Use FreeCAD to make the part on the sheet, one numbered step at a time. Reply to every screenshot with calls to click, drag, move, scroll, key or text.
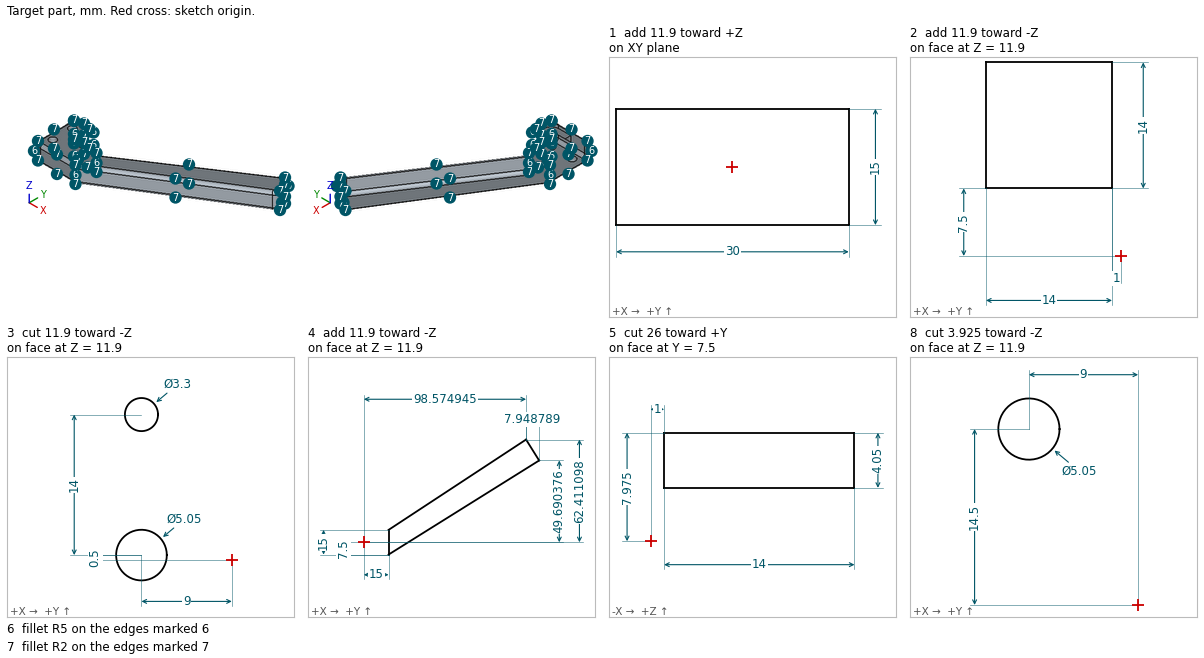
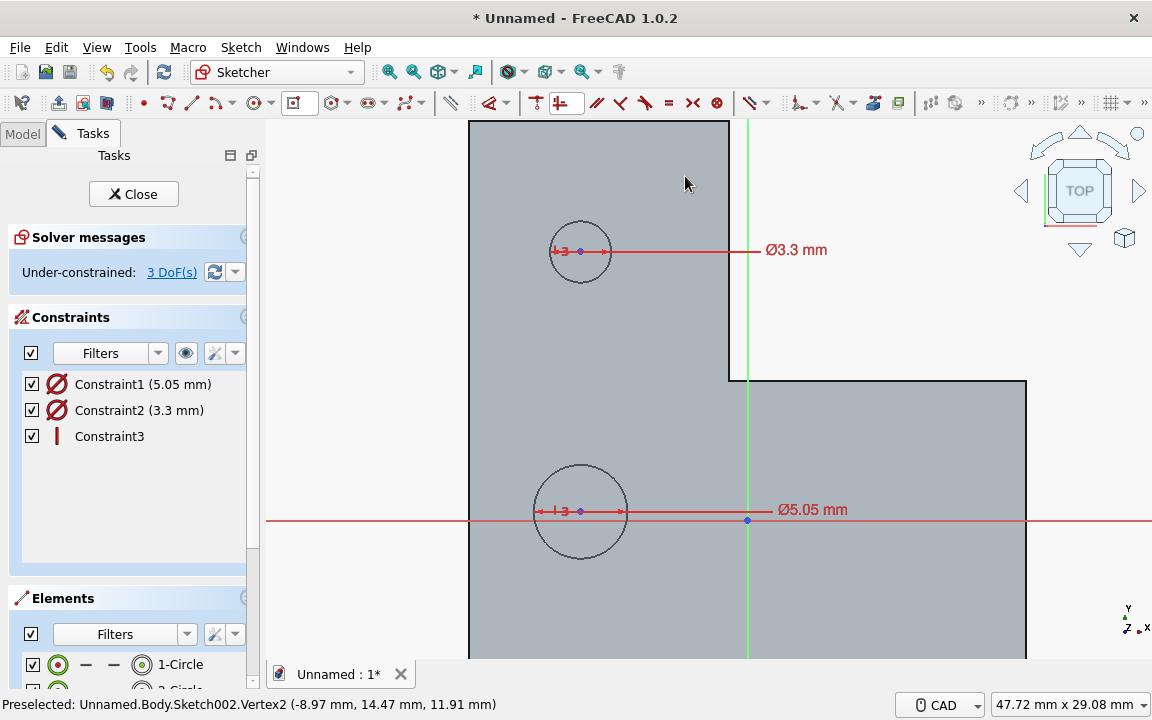
click(490, 104)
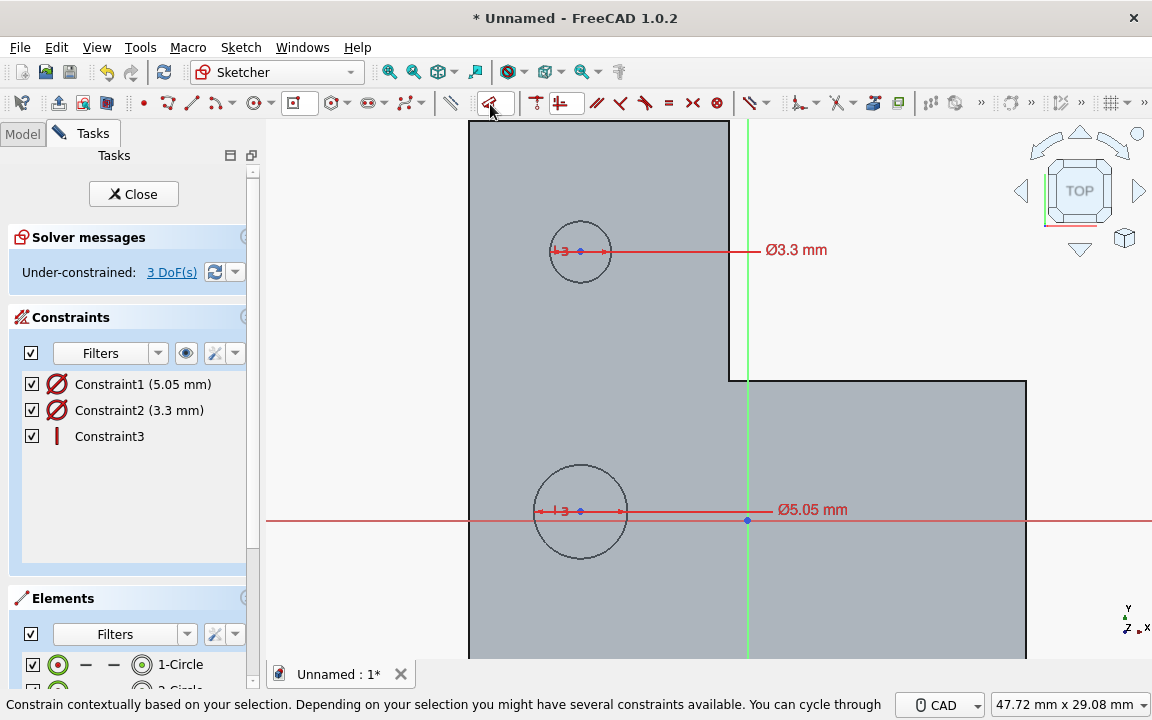
click(581, 512)
click(664, 555)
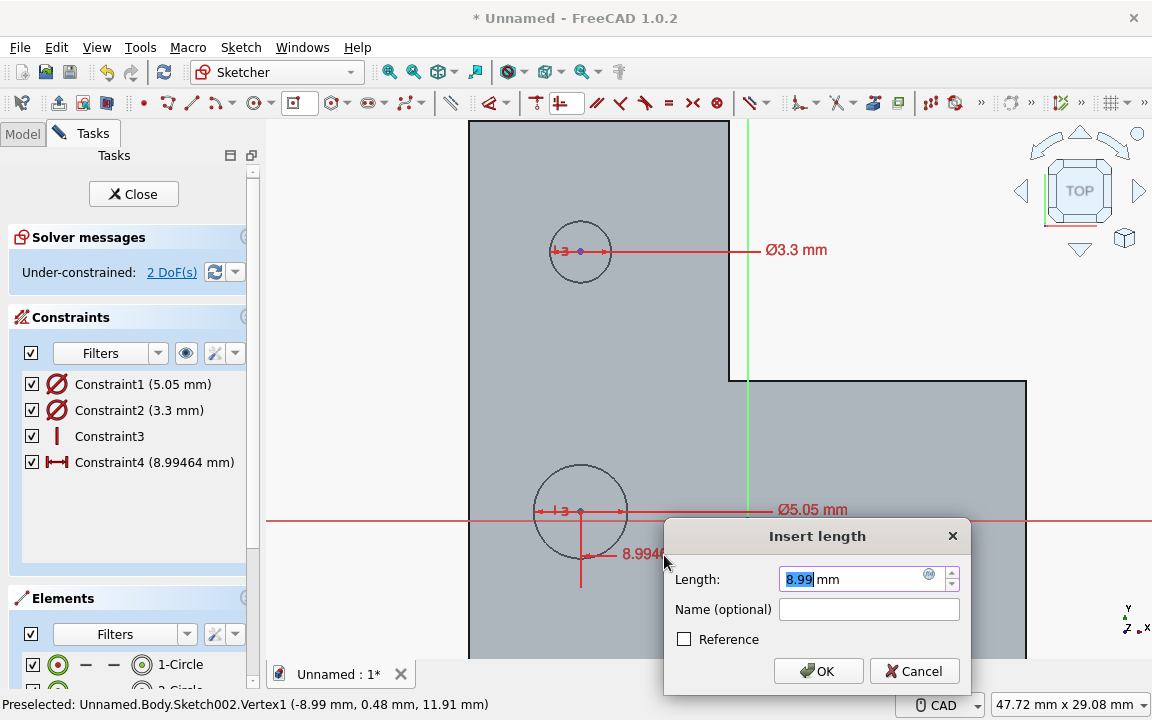
text(9)
key(Return)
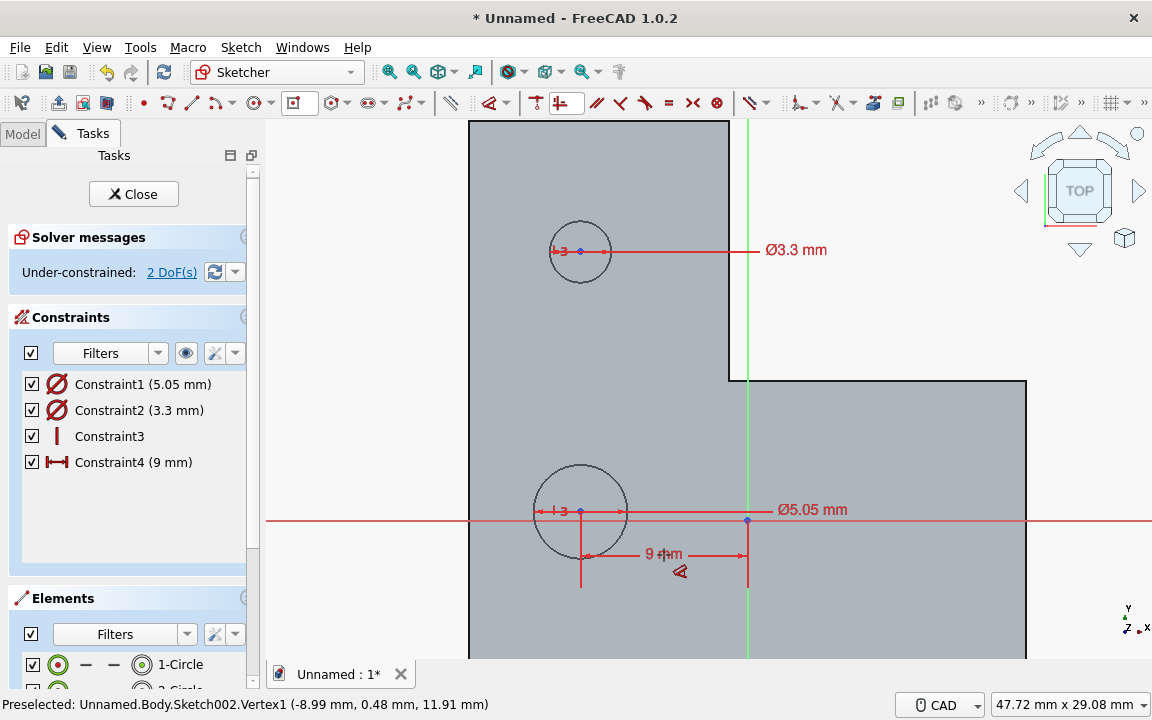
scroll(581, 512, up, 8)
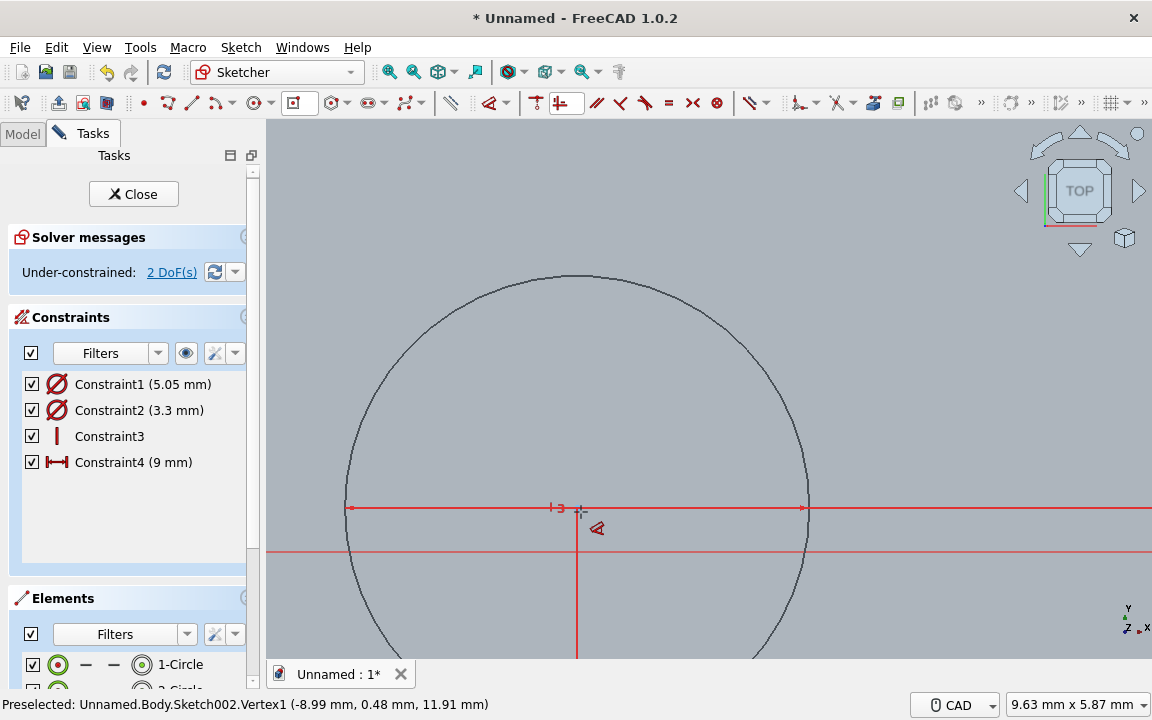
click(577, 508)
click(543, 530)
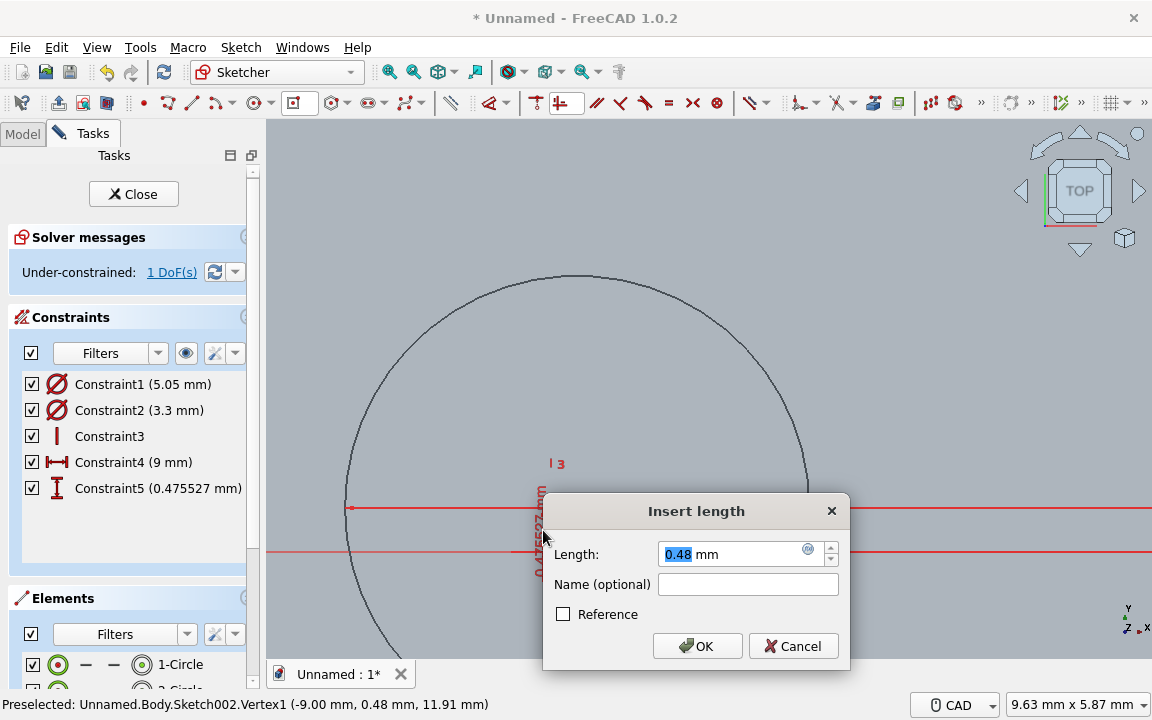
text(0.5)
key(Return)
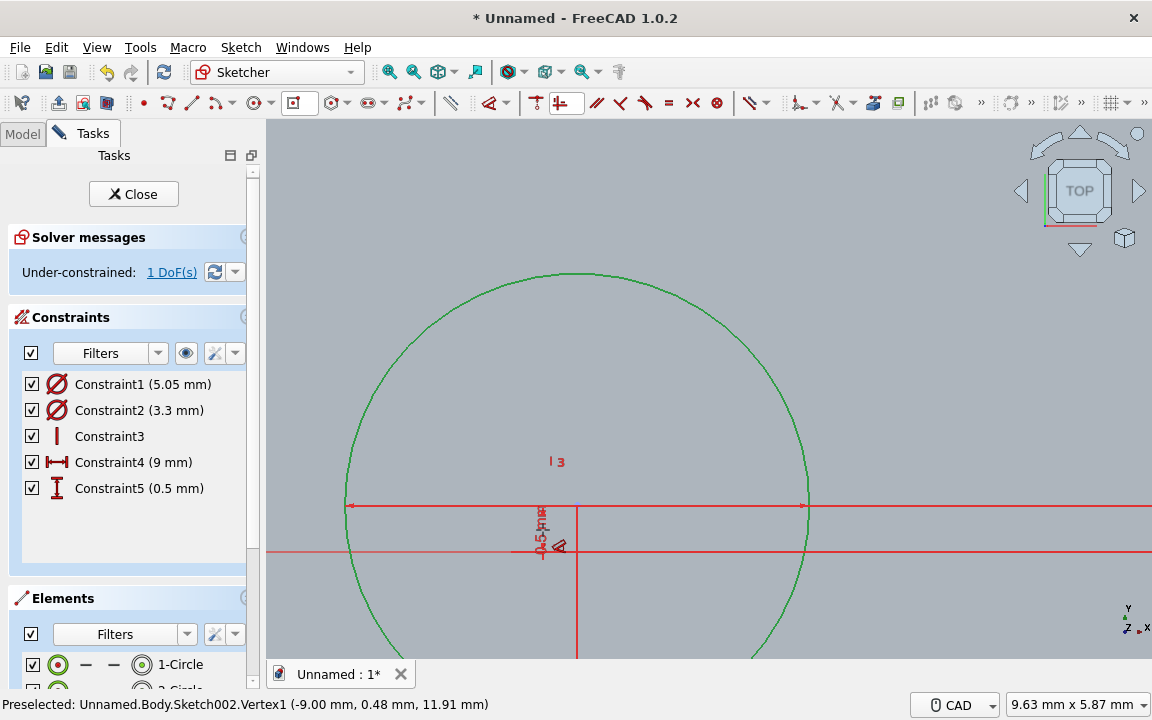
scroll(581, 512, down, 8)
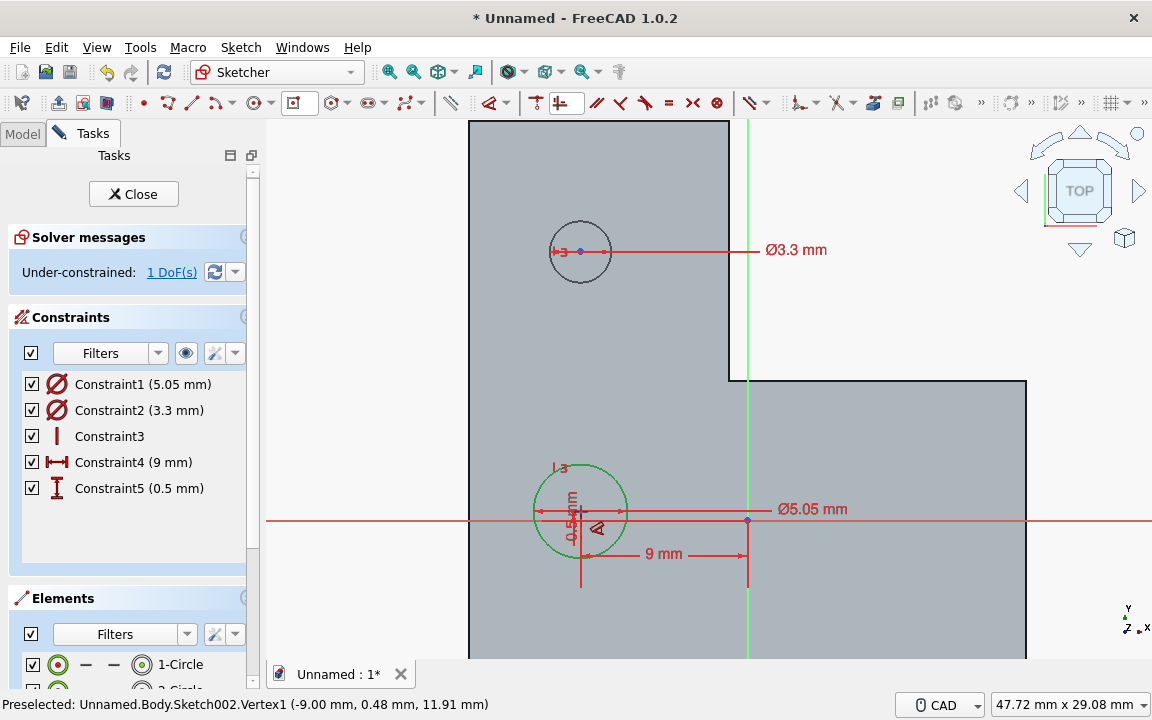
click(581, 511)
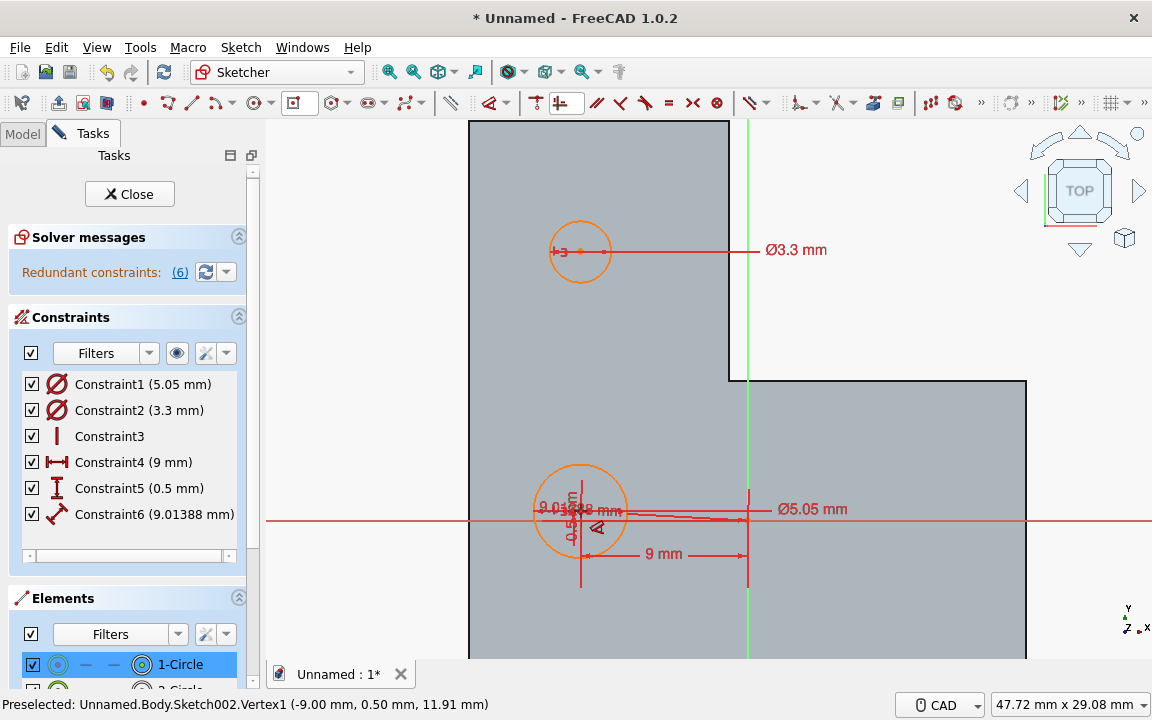
click(581, 252)
click(547, 382)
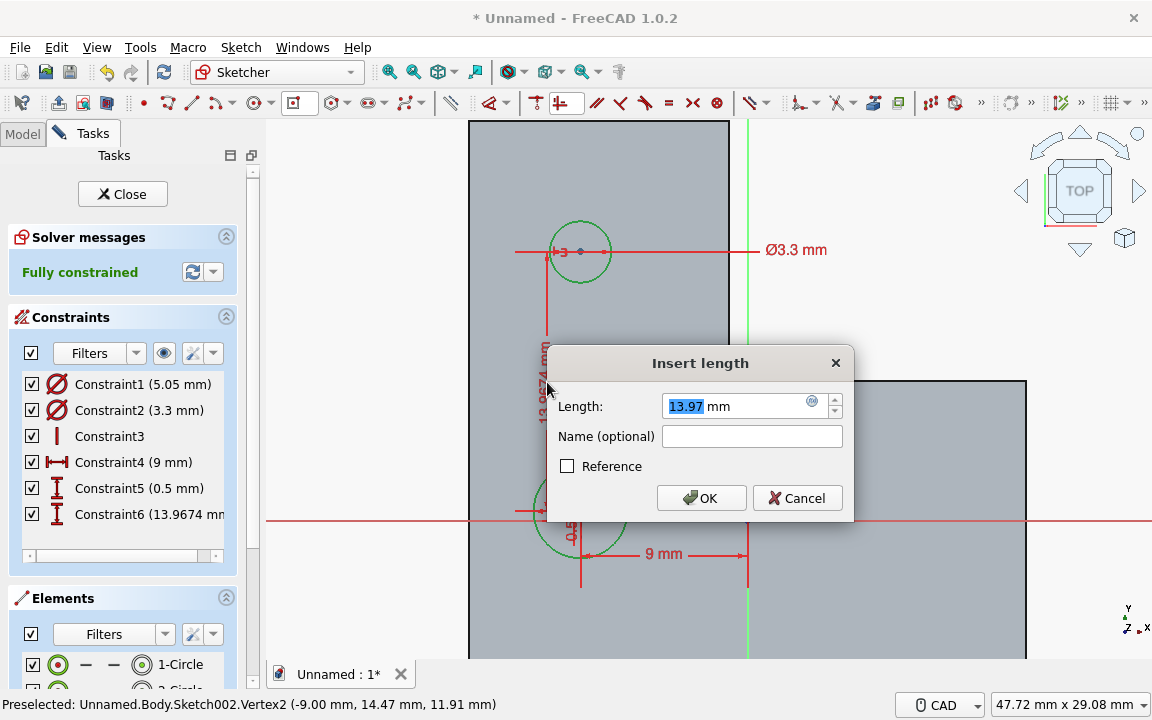
text(14)
key(Return)
key(Escape)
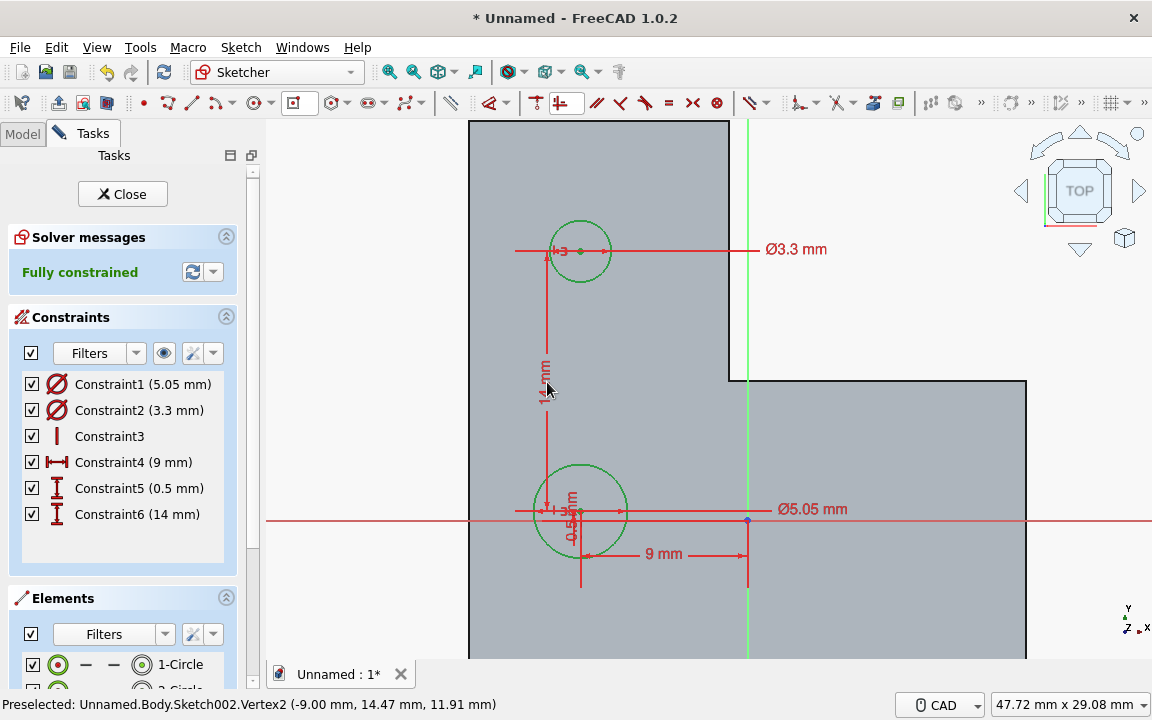
click(123, 194)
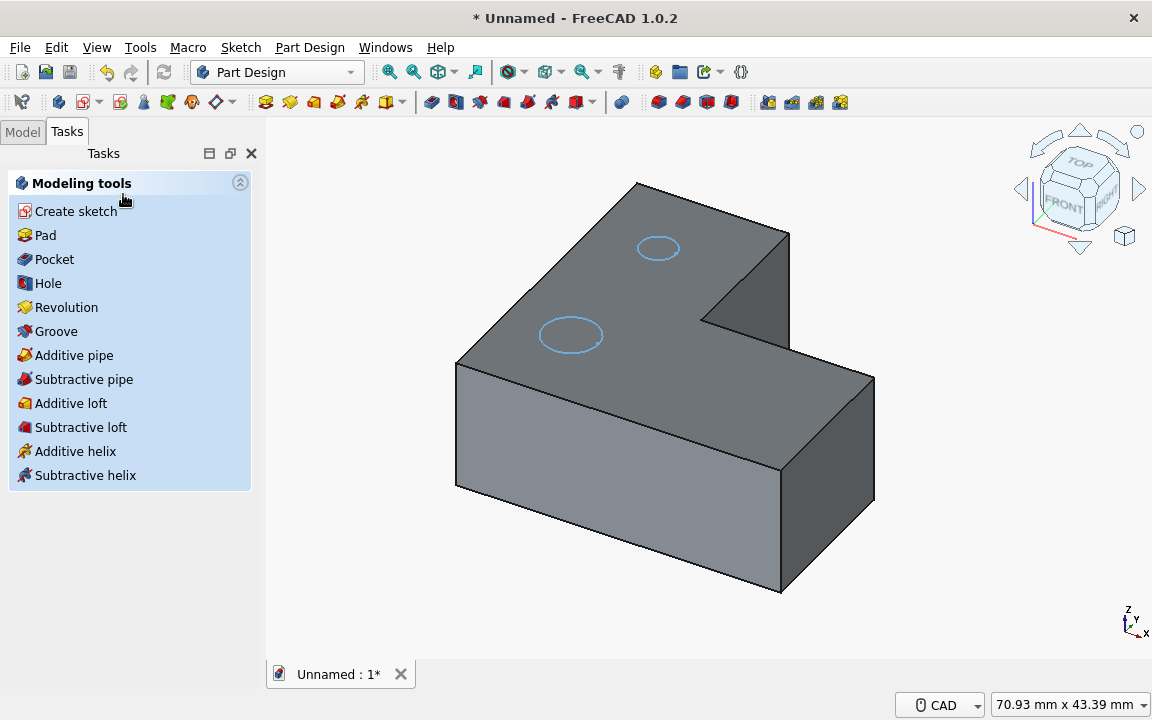
click(432, 102)